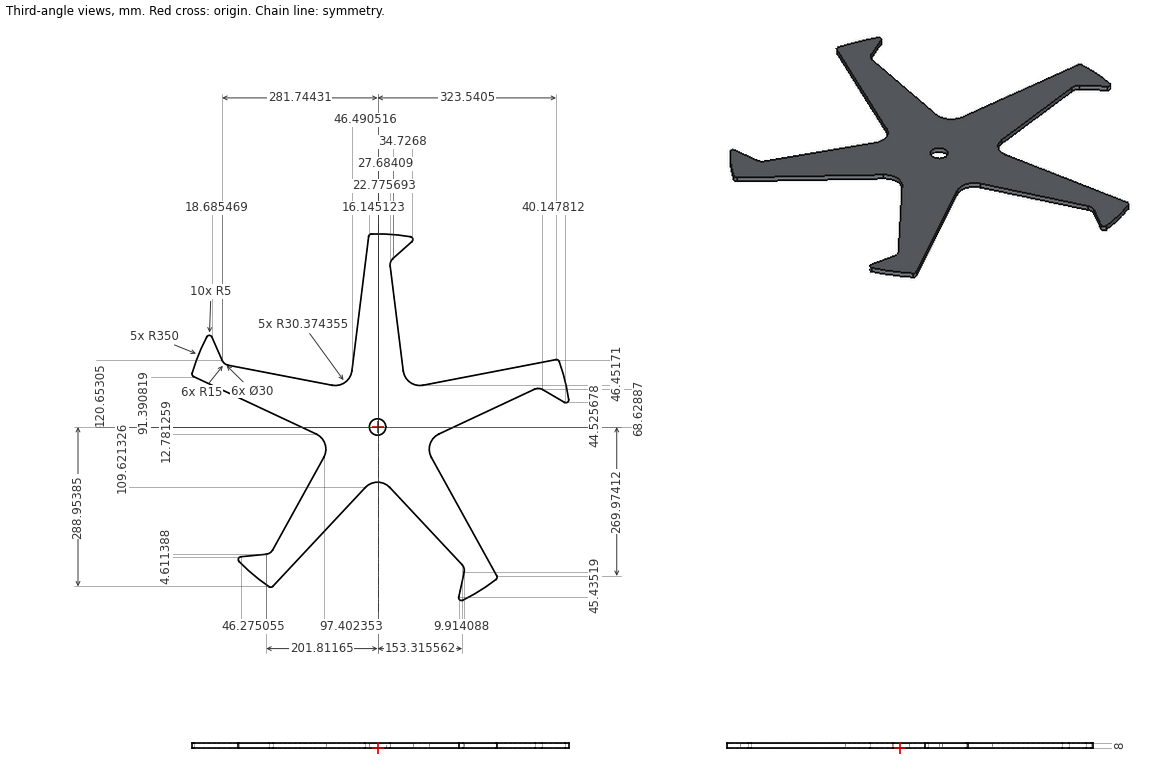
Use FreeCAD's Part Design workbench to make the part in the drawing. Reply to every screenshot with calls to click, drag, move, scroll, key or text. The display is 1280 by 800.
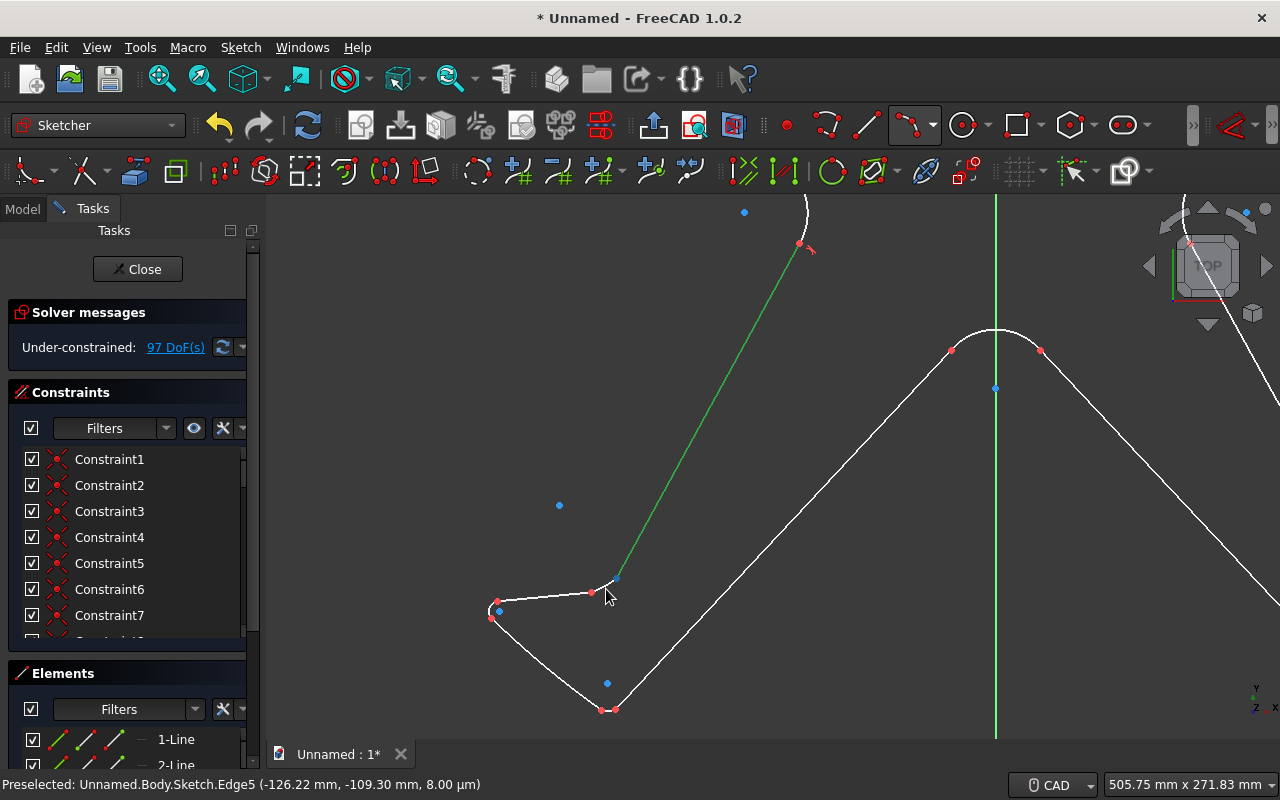
click(605, 586)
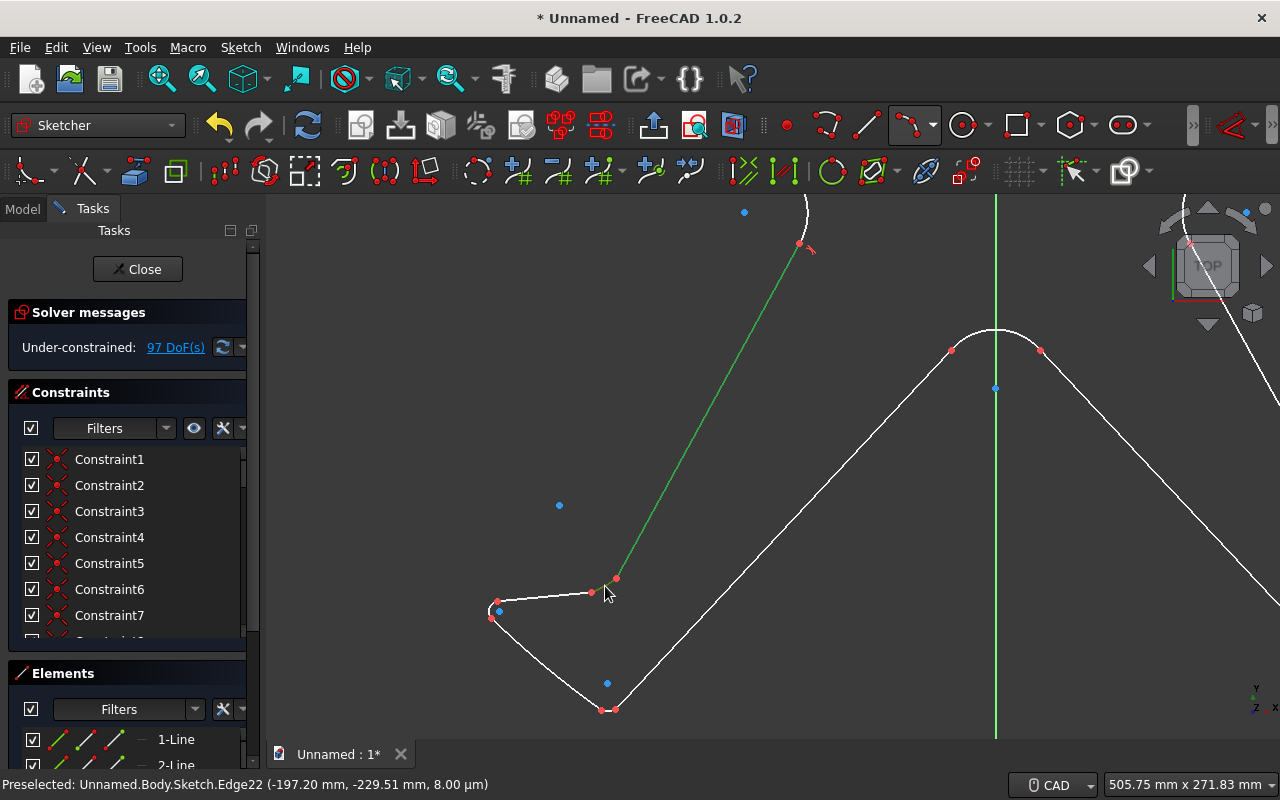
key(t)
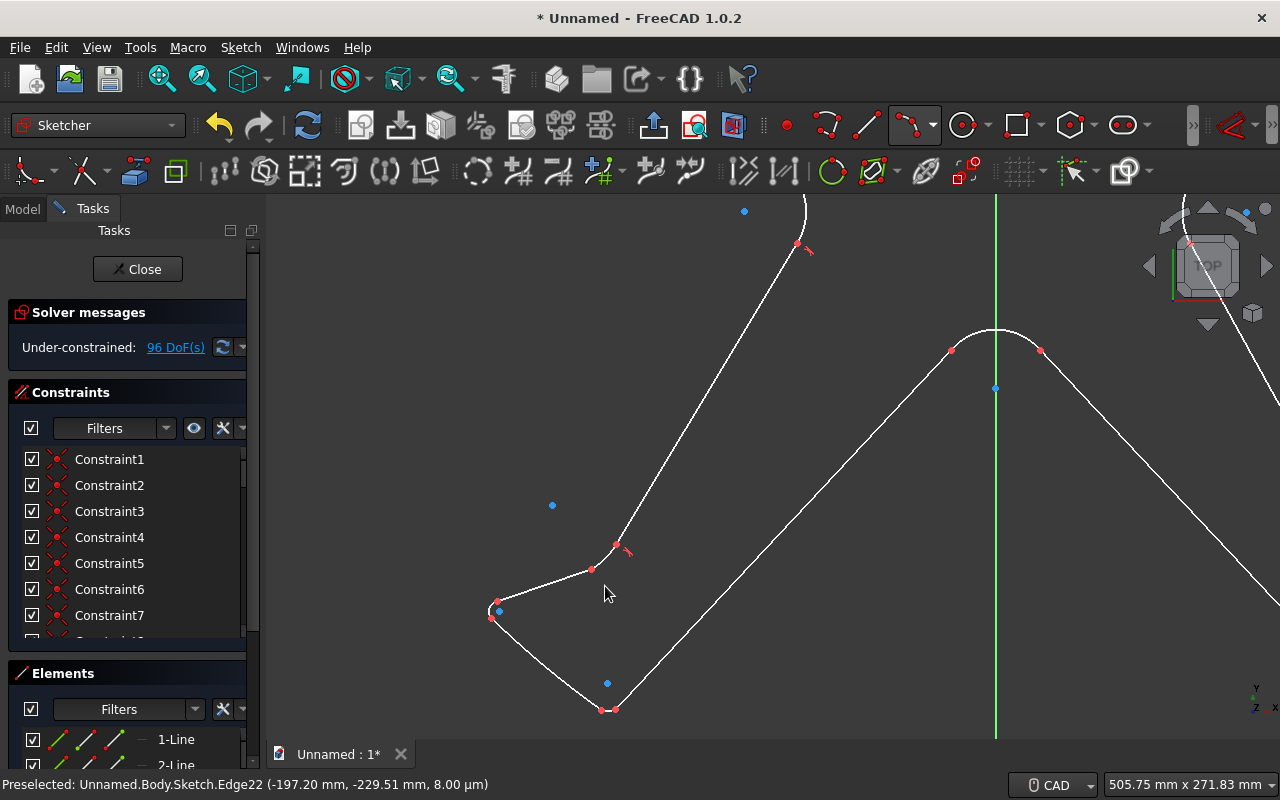
click(563, 579)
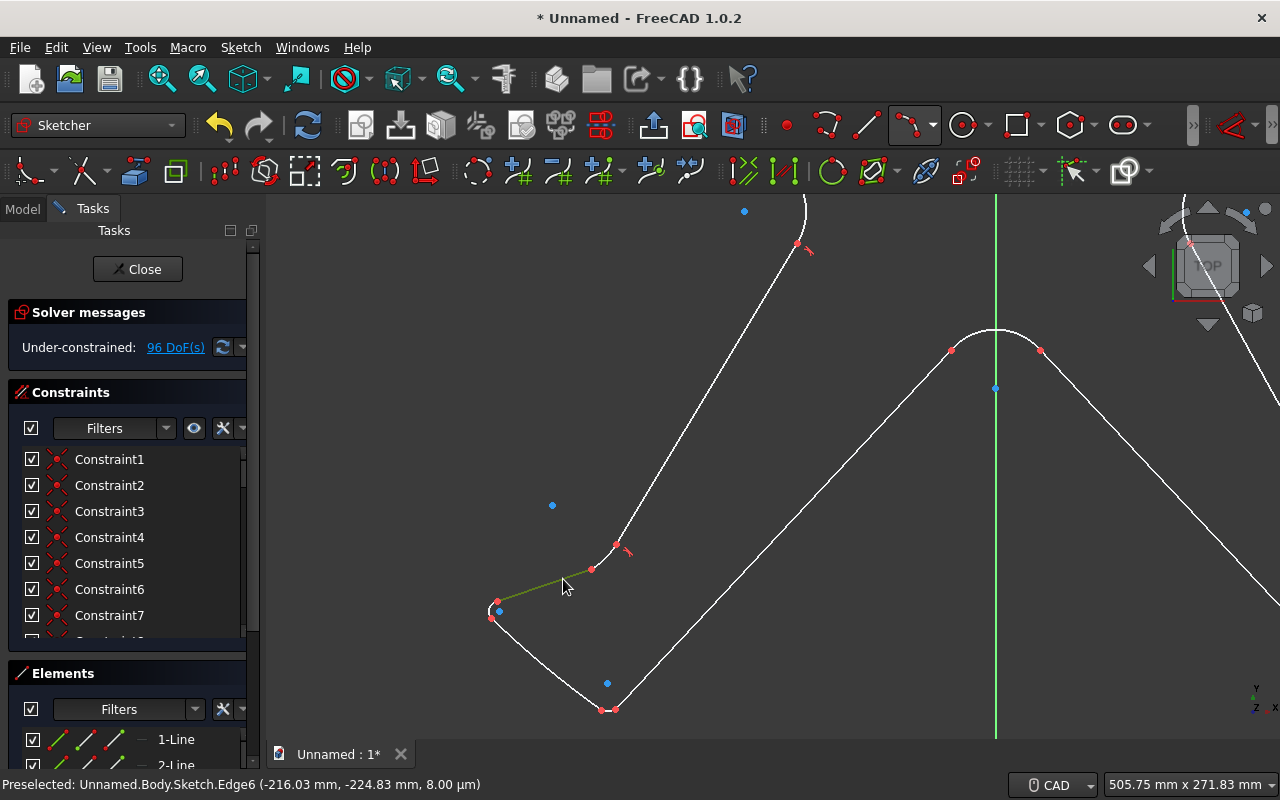
scroll(600, 563, up, 2)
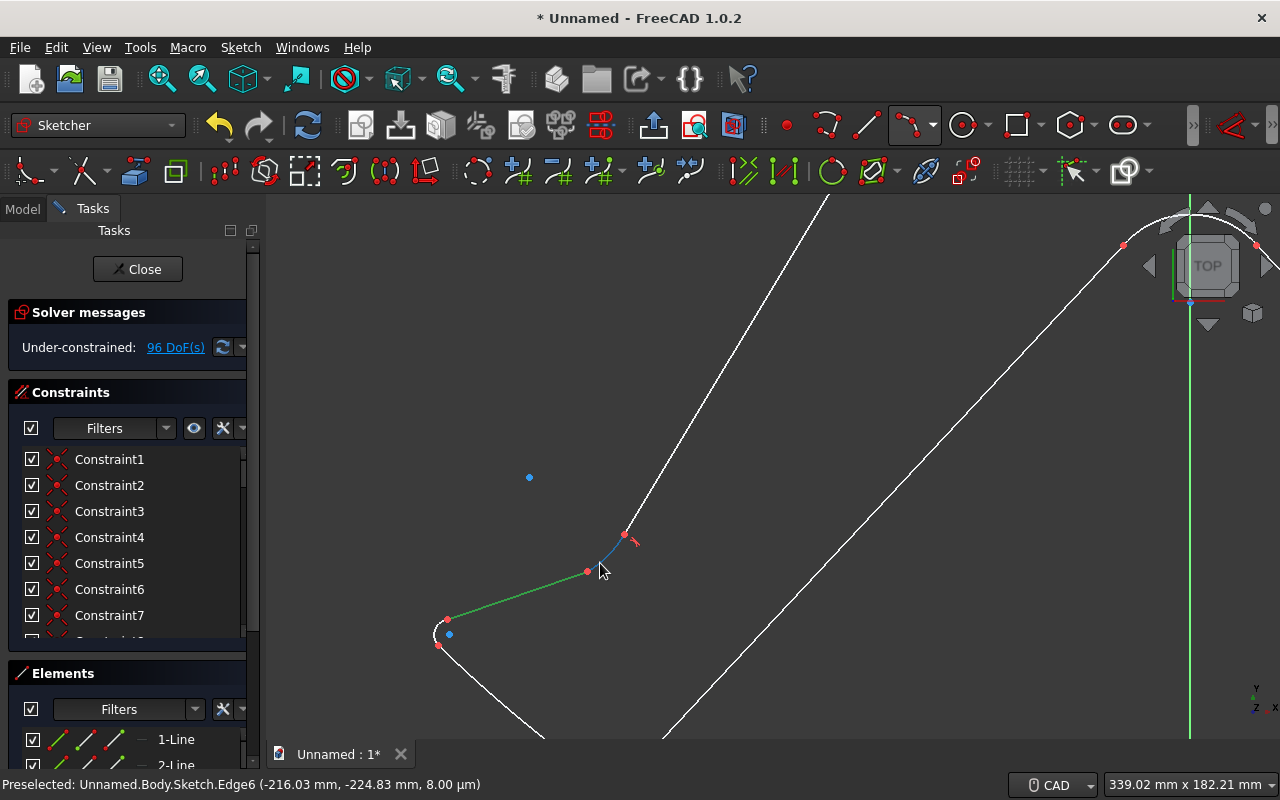
click(600, 563)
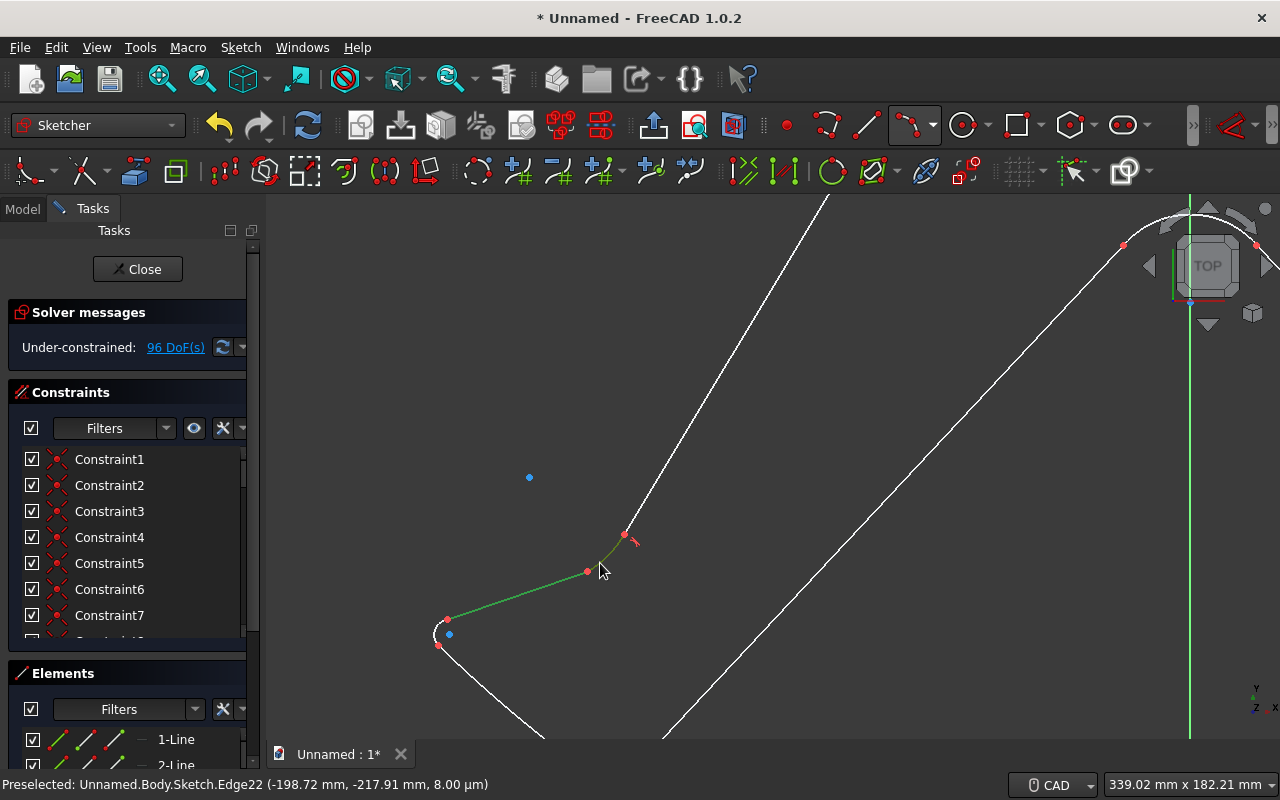
key(t)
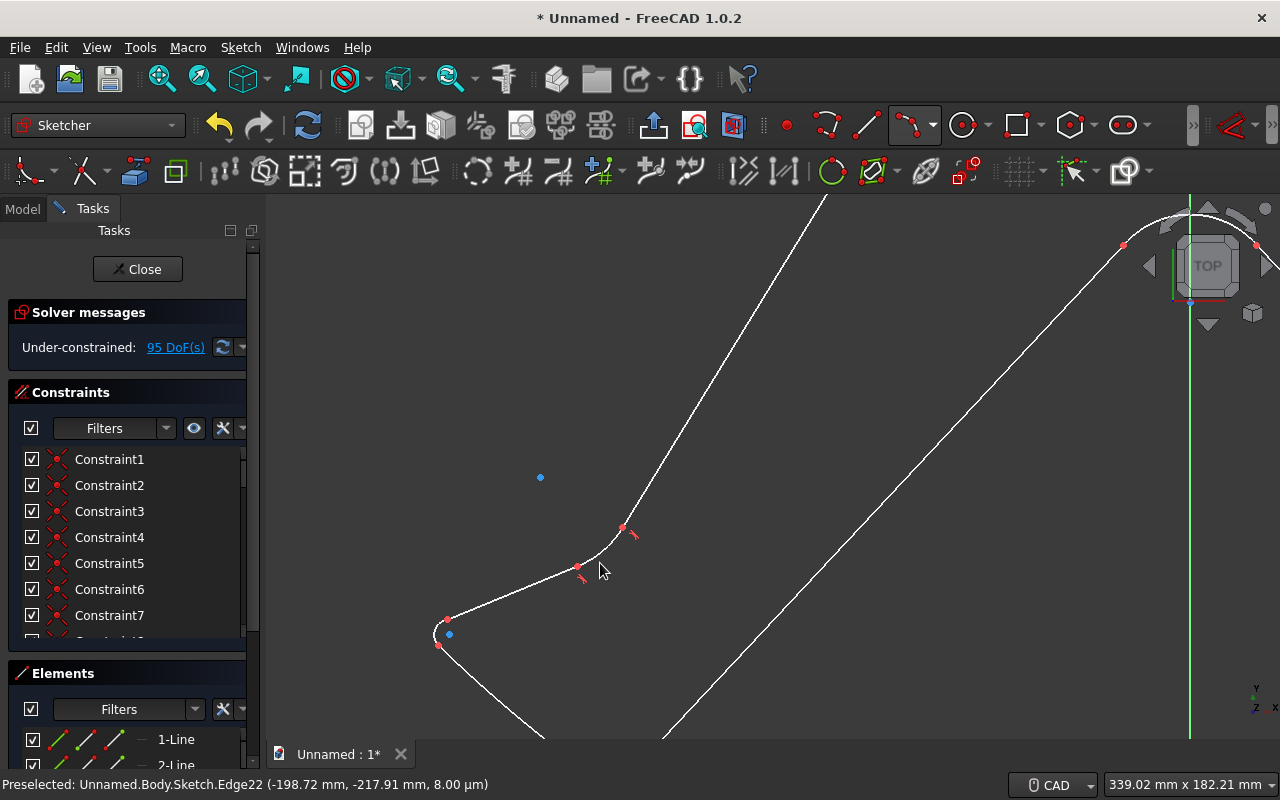
scroll(605, 586, down, 9)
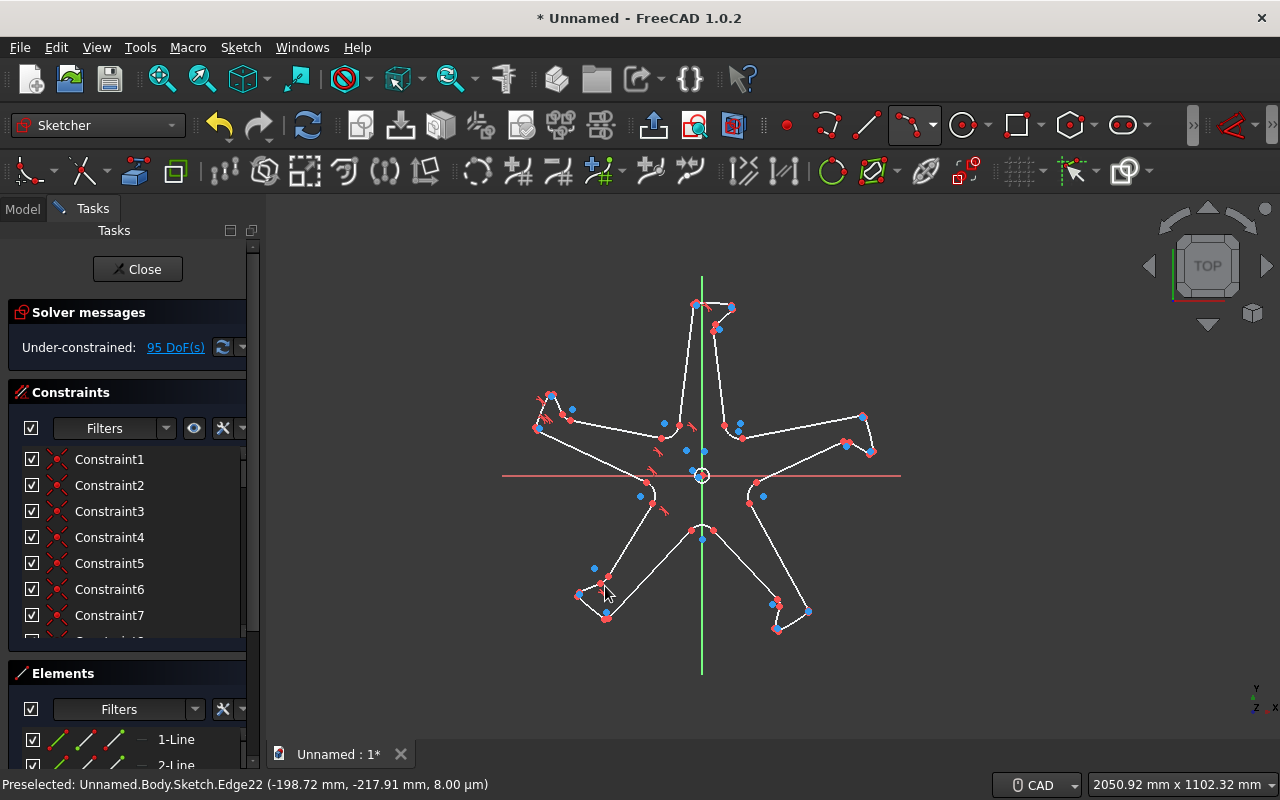
scroll(594, 586, up, 4)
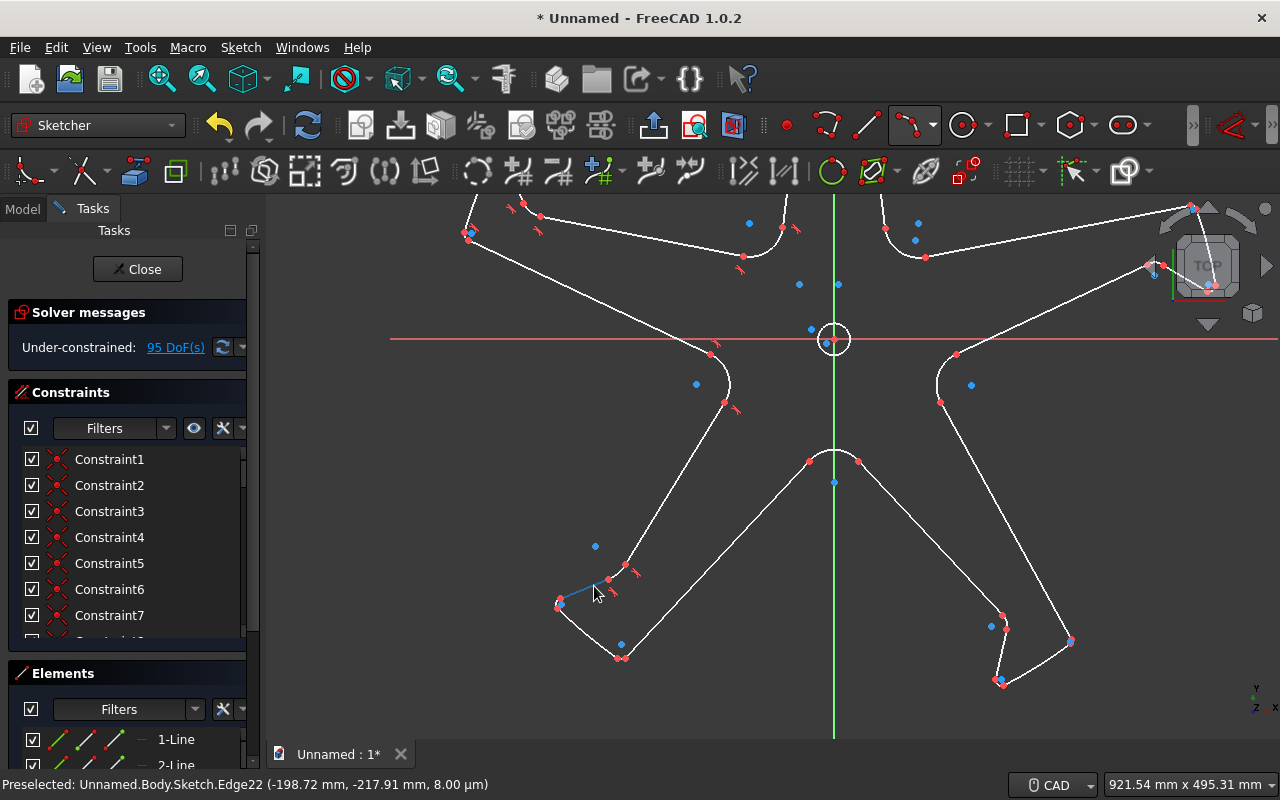
click(594, 585)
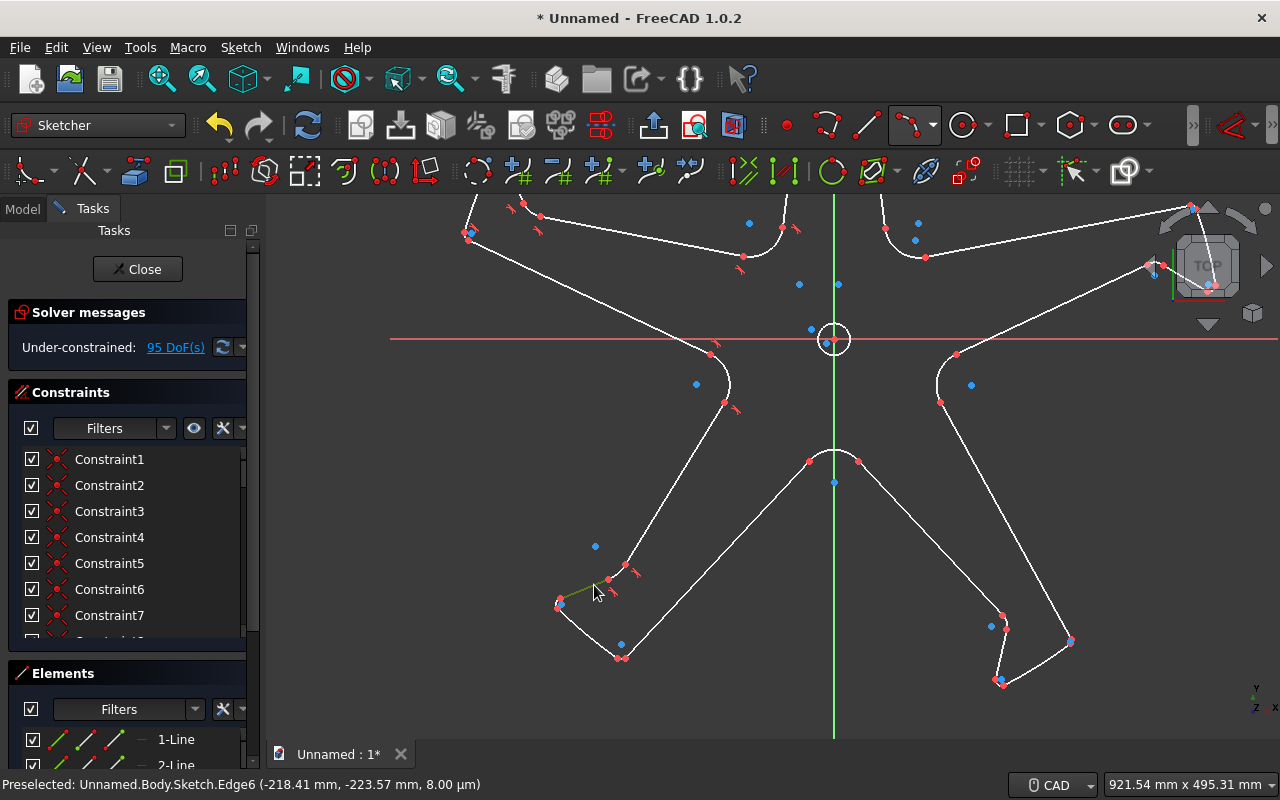
scroll(556, 603, up, 5)